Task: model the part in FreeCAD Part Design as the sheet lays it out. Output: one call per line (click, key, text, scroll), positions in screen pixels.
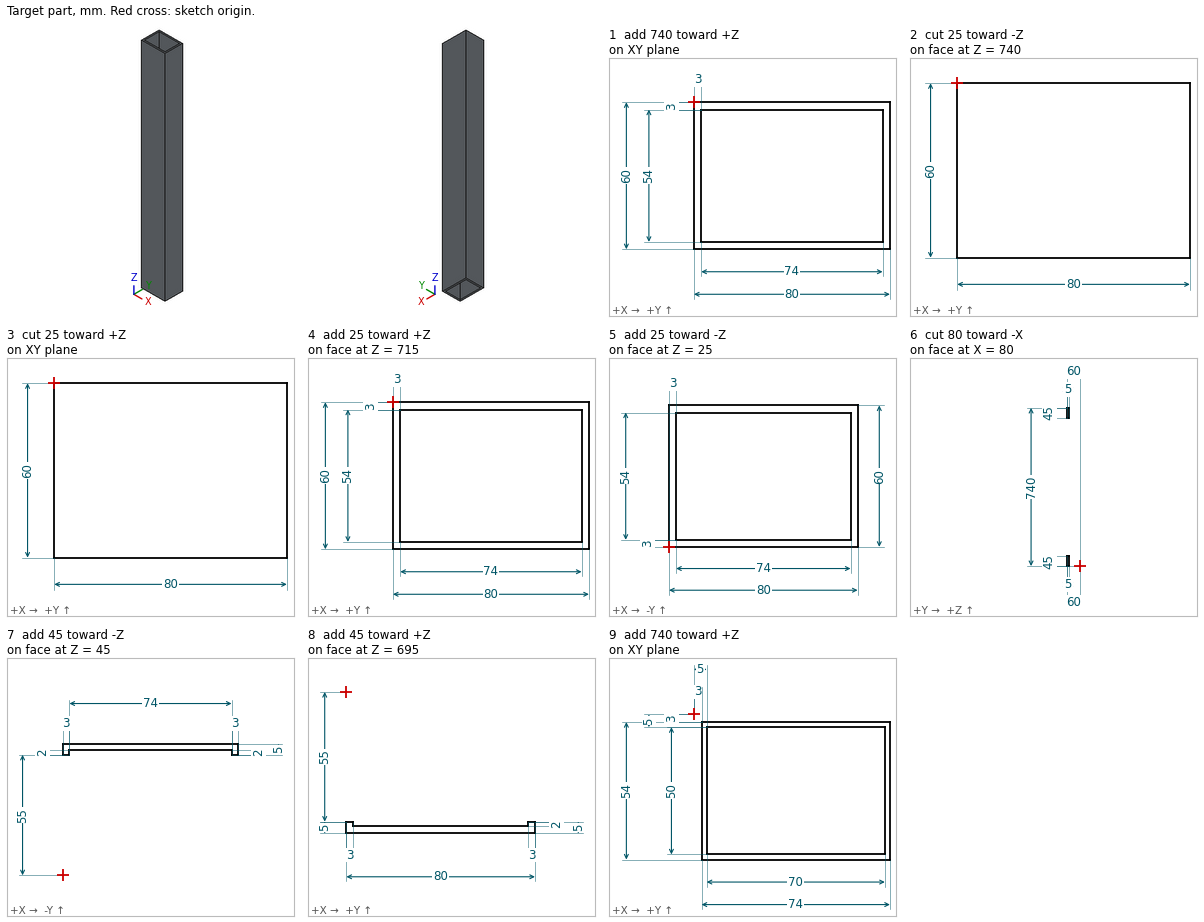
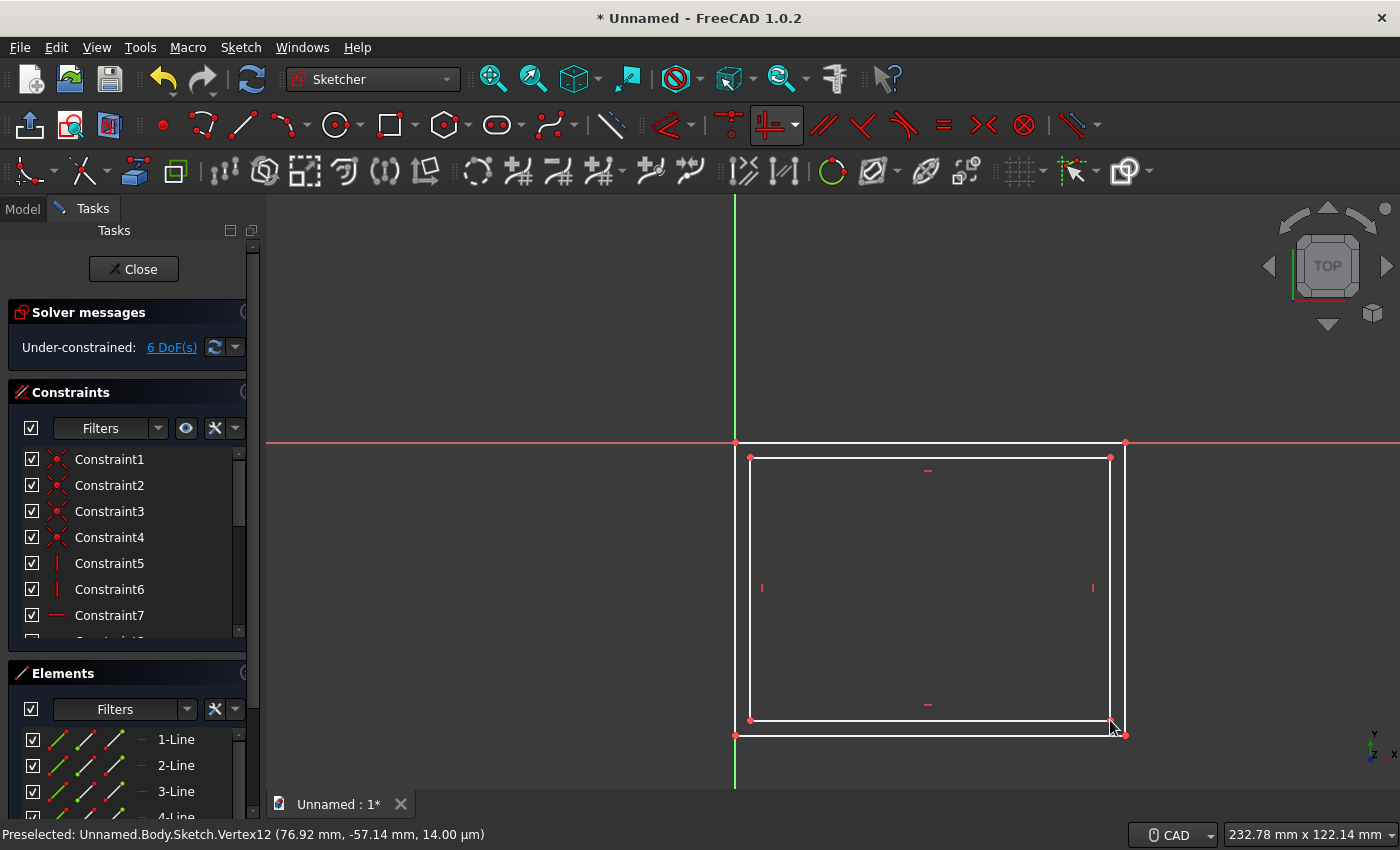
key(d)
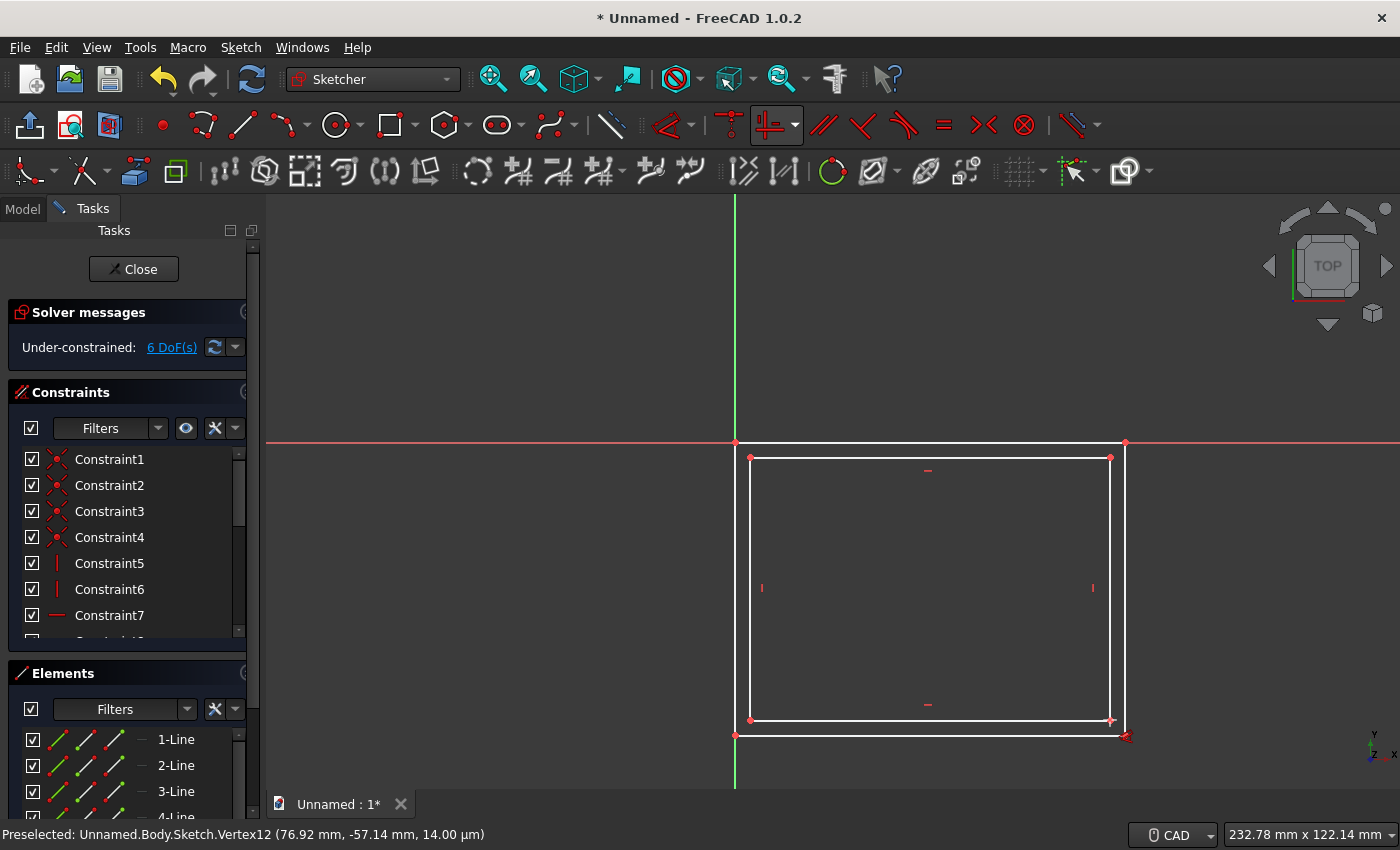
click(735, 531)
click(701, 589)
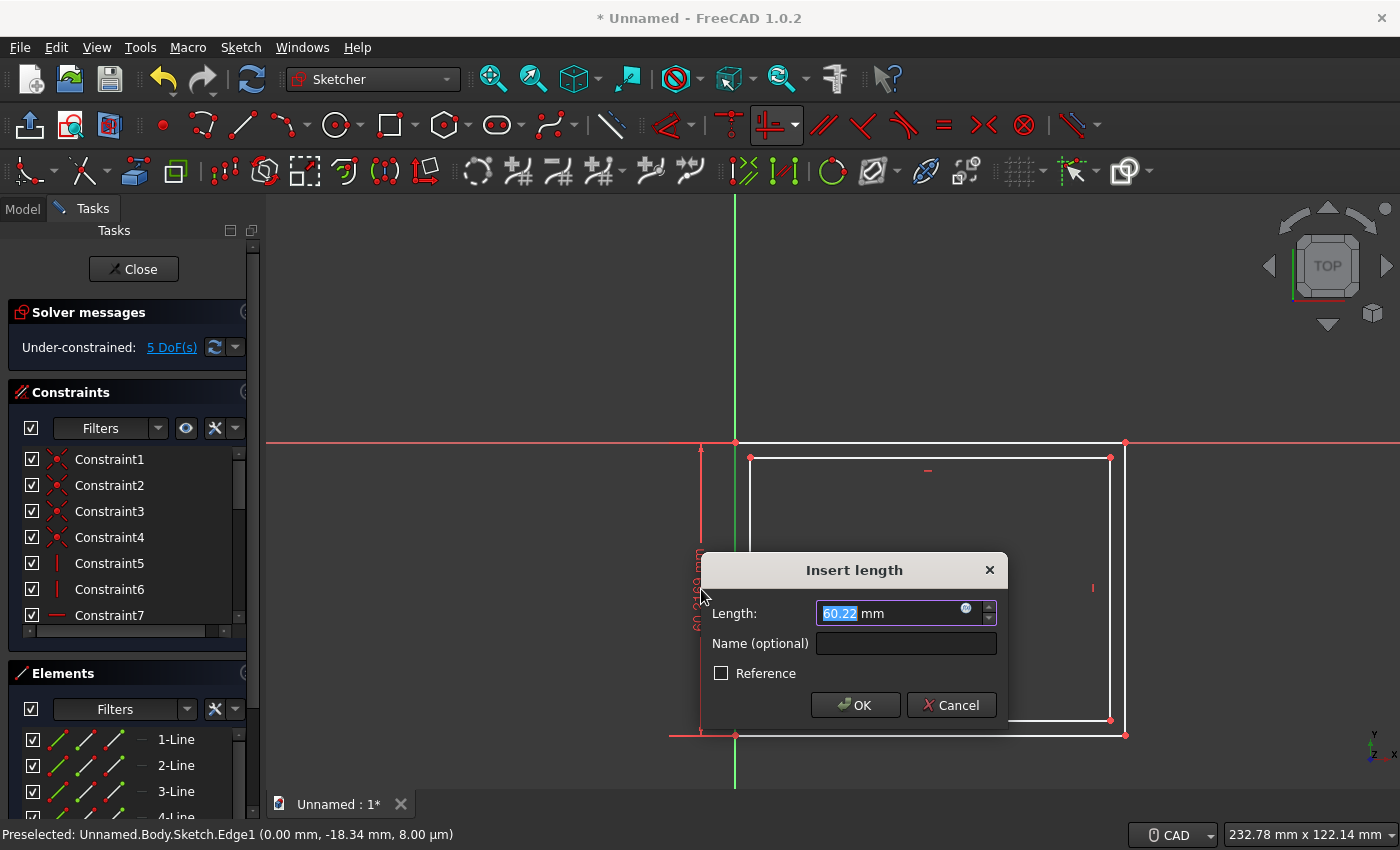
text(60)
key(Return)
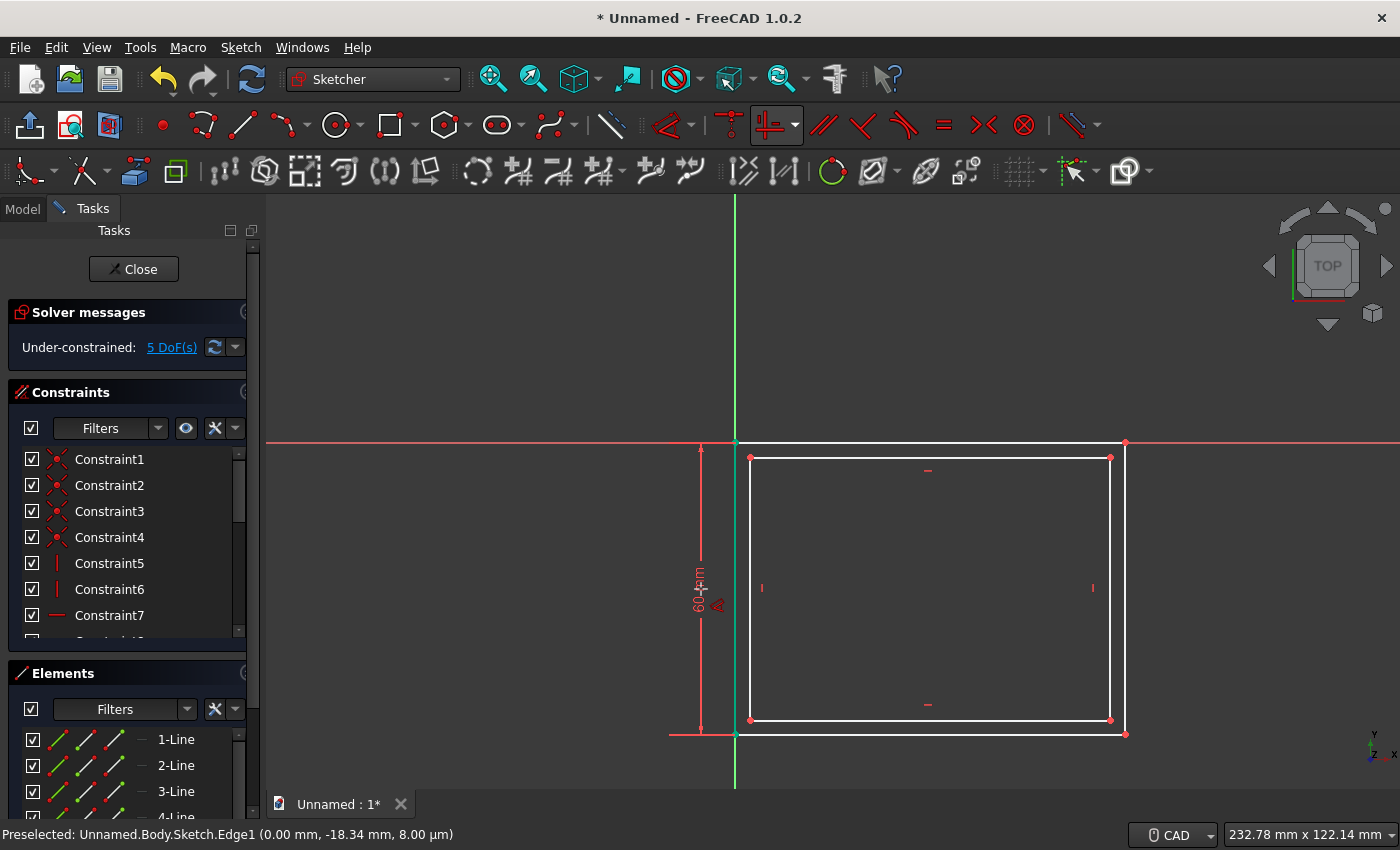
click(852, 735)
click(930, 701)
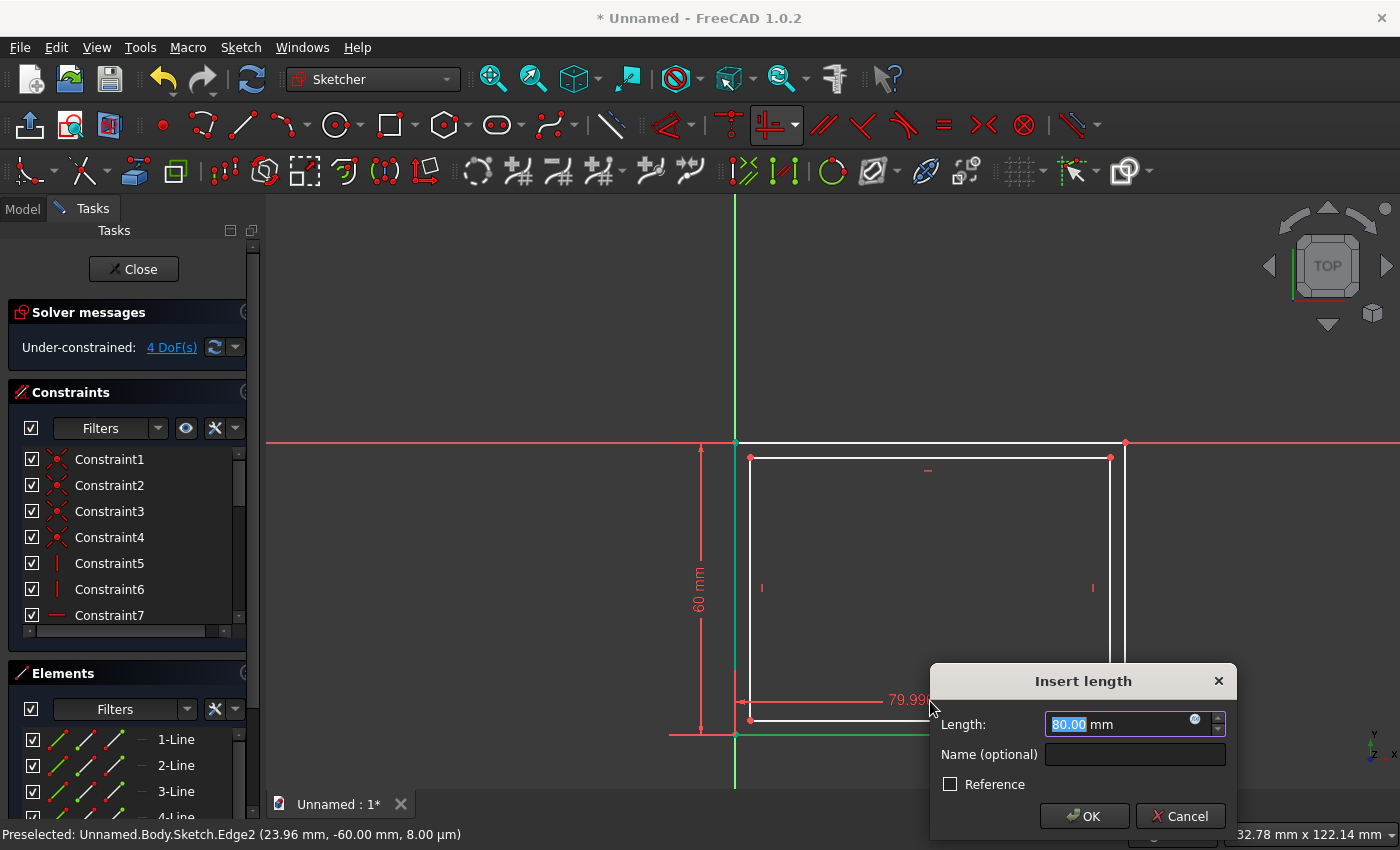
text(80)
key(Return)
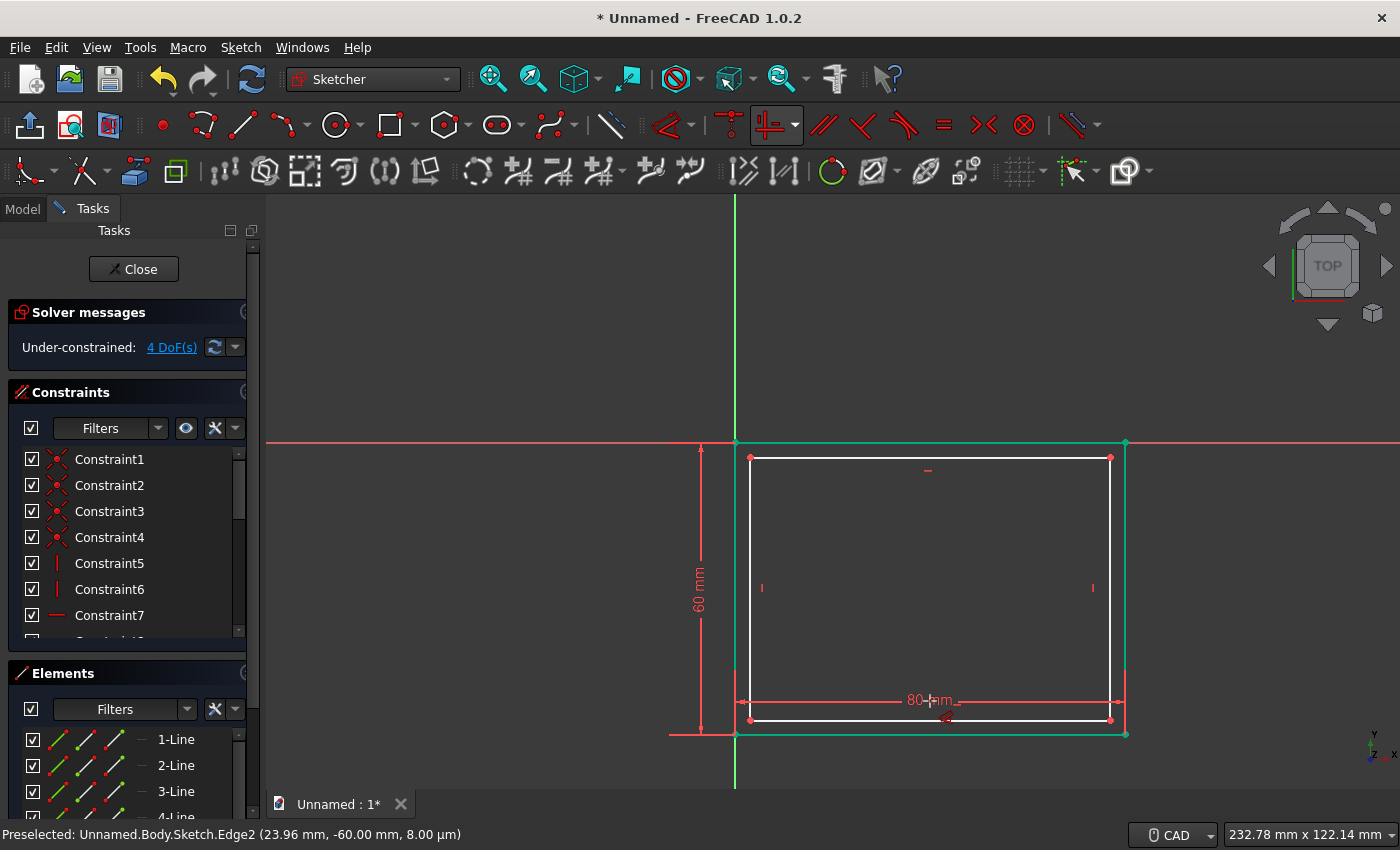
click(750, 537)
click(716, 529)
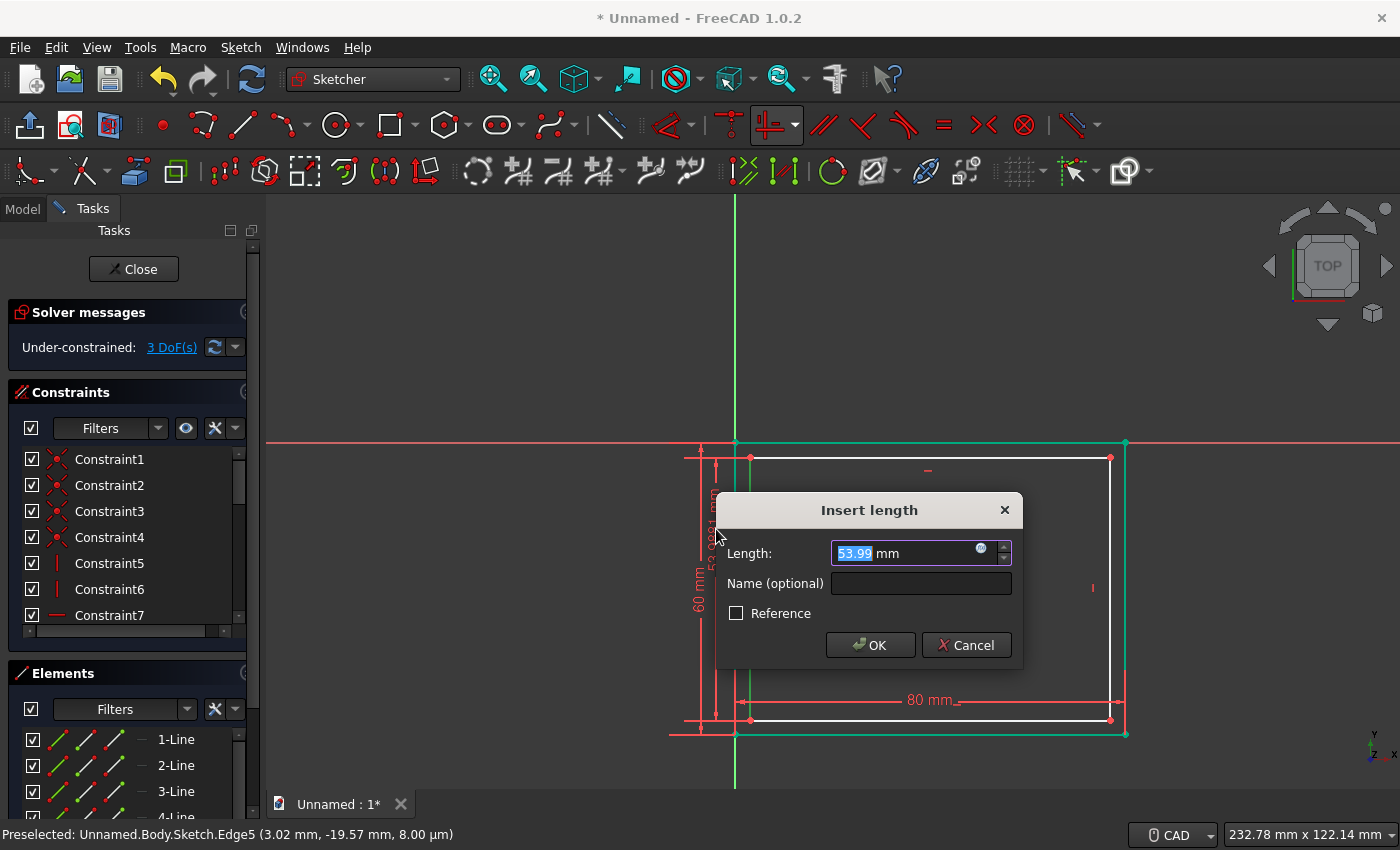
text(54)
key(Return)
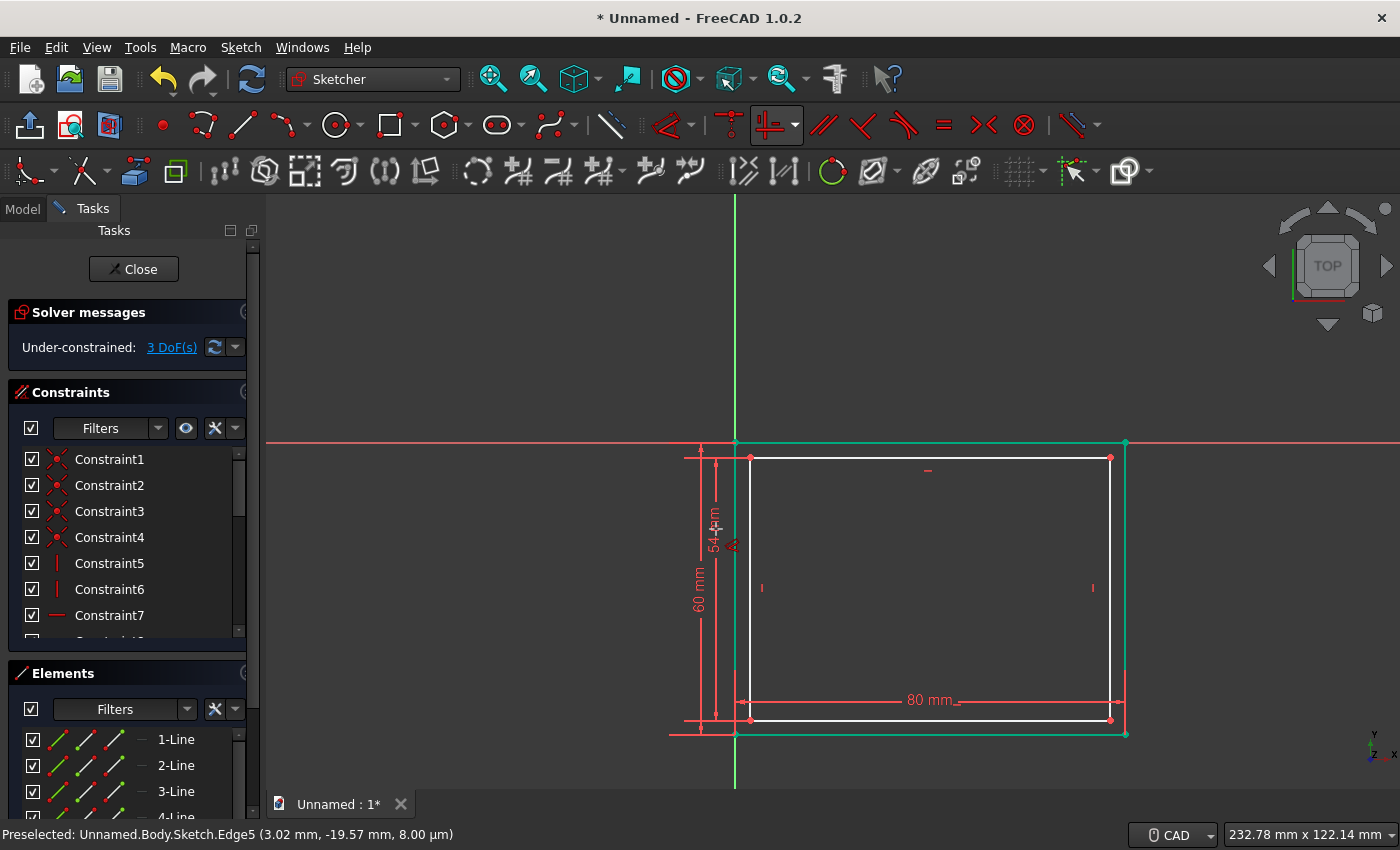
click(858, 721)
click(930, 755)